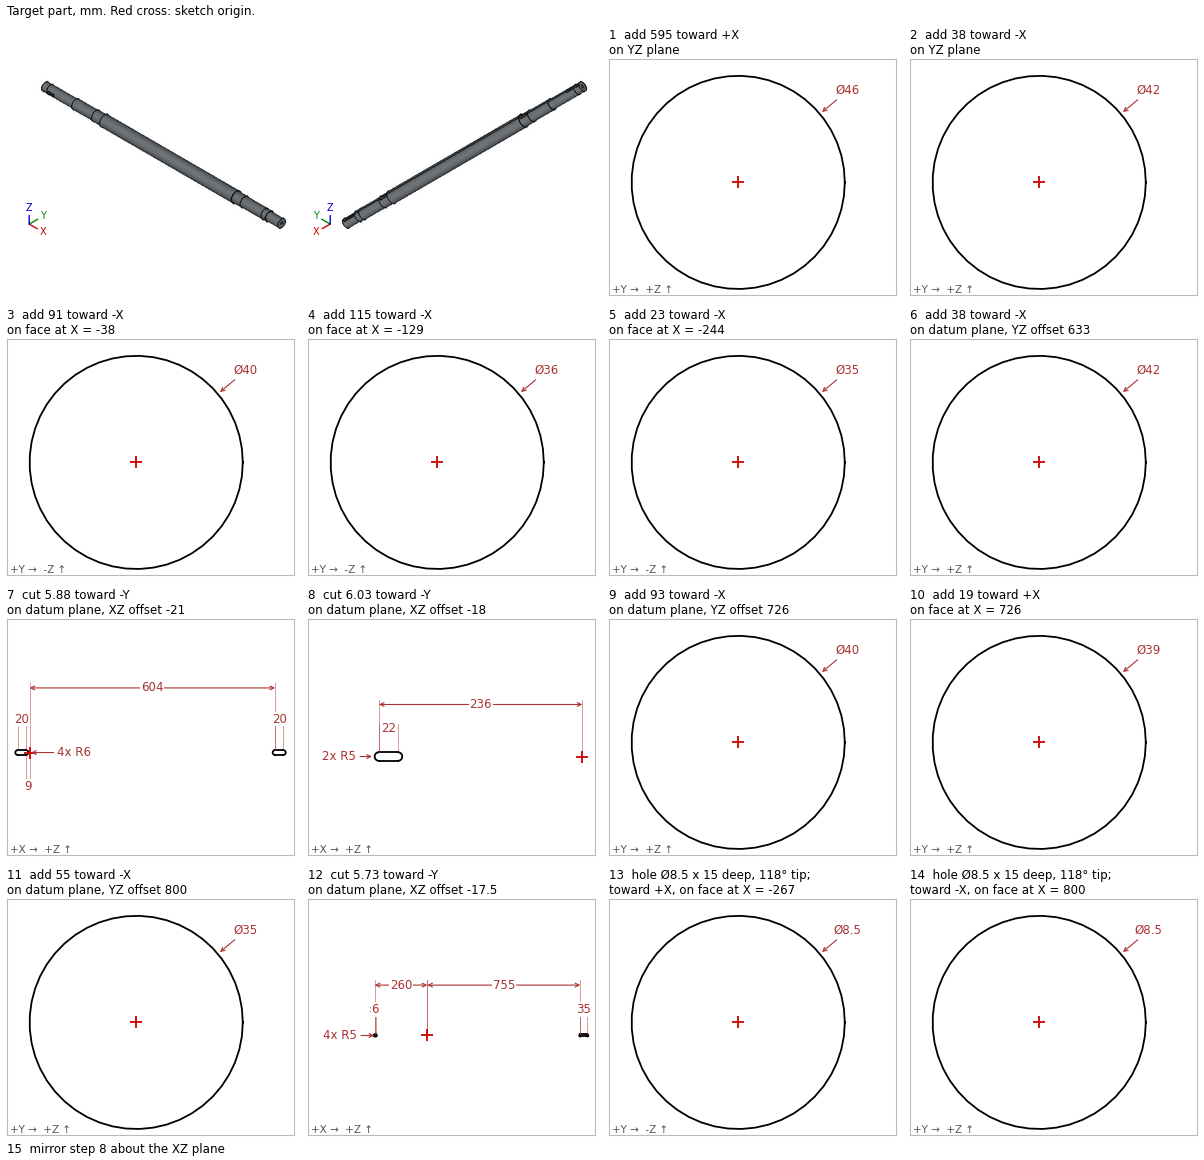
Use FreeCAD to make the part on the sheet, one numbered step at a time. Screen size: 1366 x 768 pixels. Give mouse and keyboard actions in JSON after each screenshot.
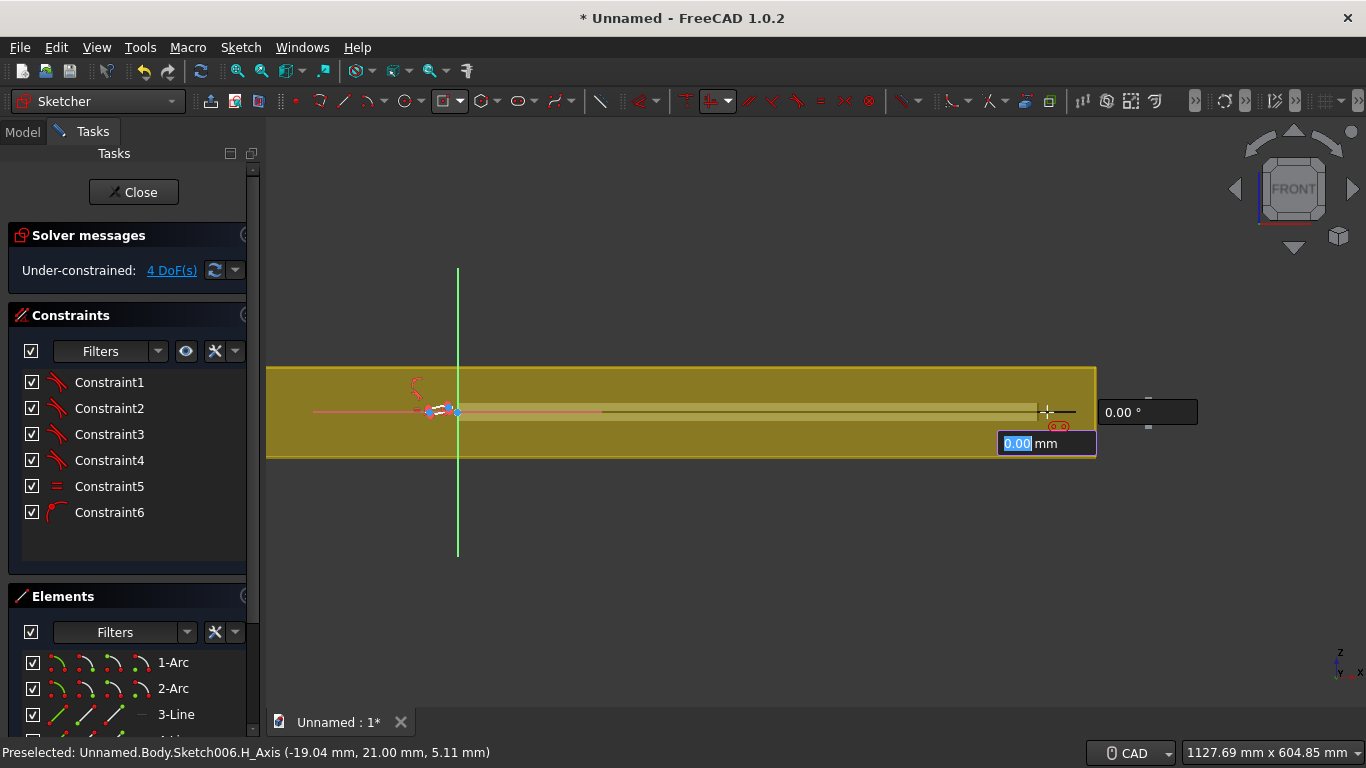
{"action": "left_click", "coordinate": [1066, 403]}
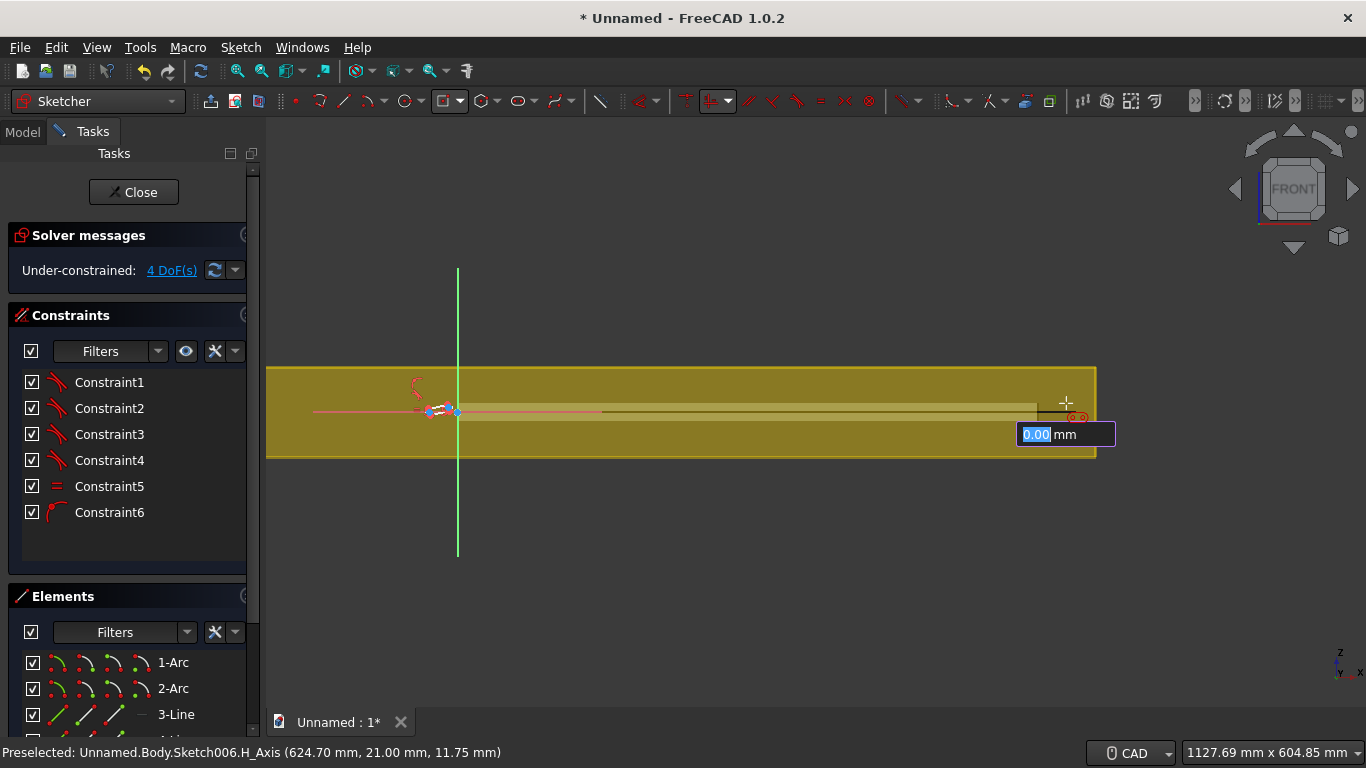
{"action": "scroll", "coordinate": [1057, 418], "scroll_direction": "up", "scroll_amount": 5}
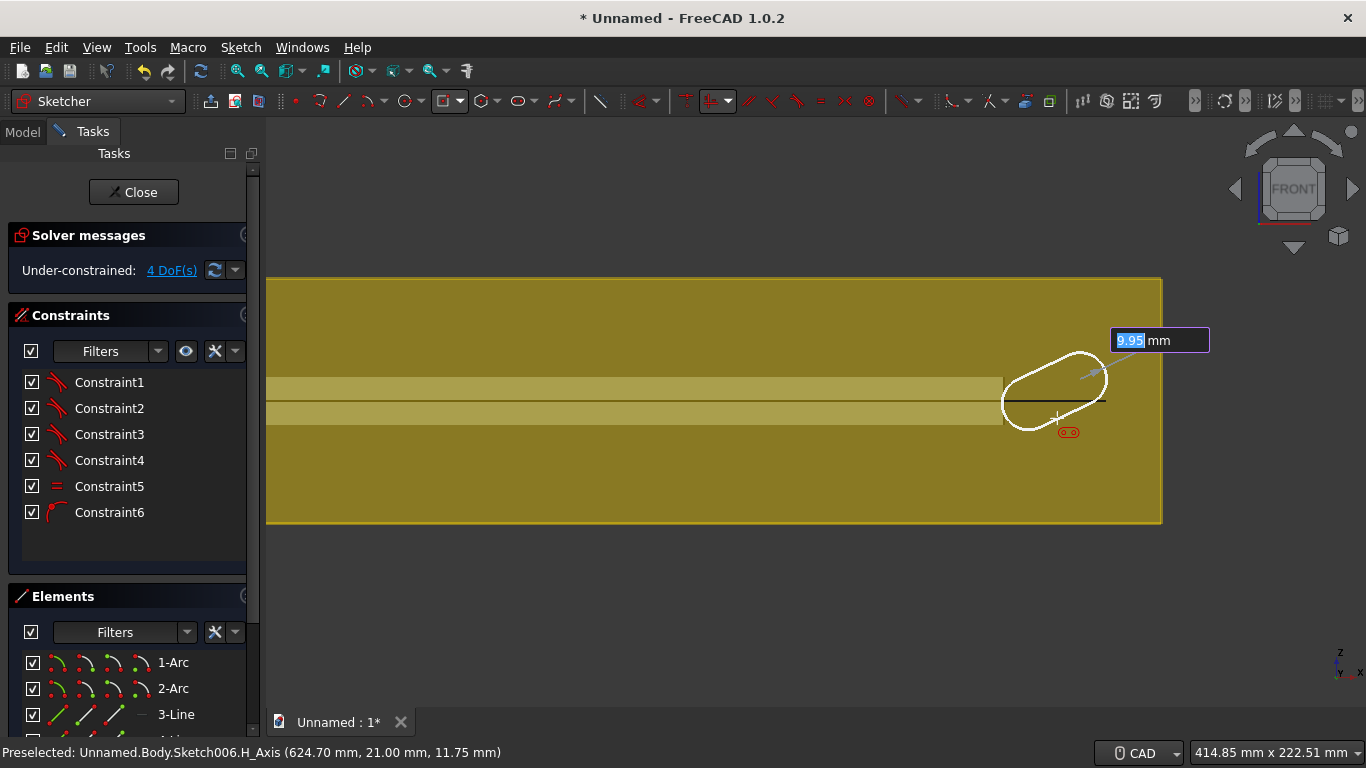
{"action": "left_click", "coordinate": [1055, 417]}
{"action": "key", "text": "Escape"}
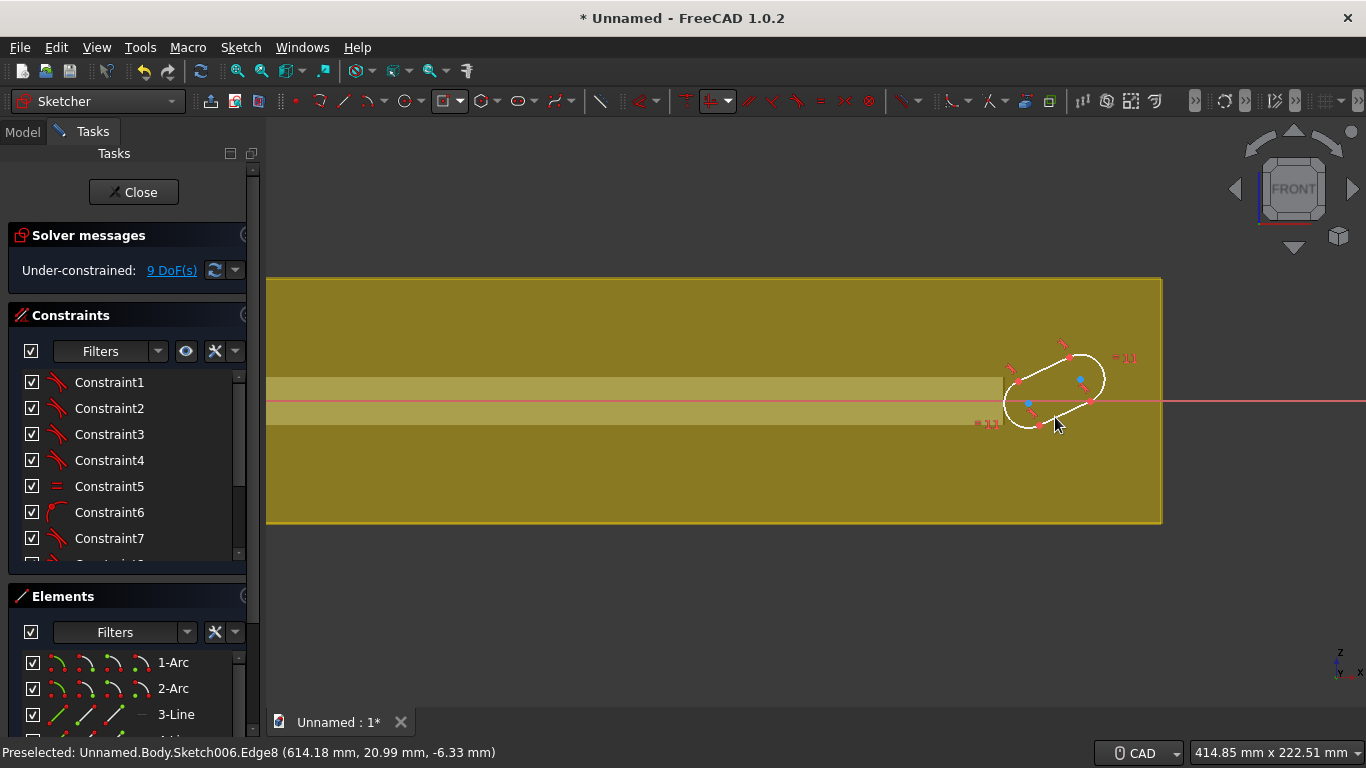
{"action": "scroll", "coordinate": [1057, 418], "scroll_direction": "down", "scroll_amount": 5}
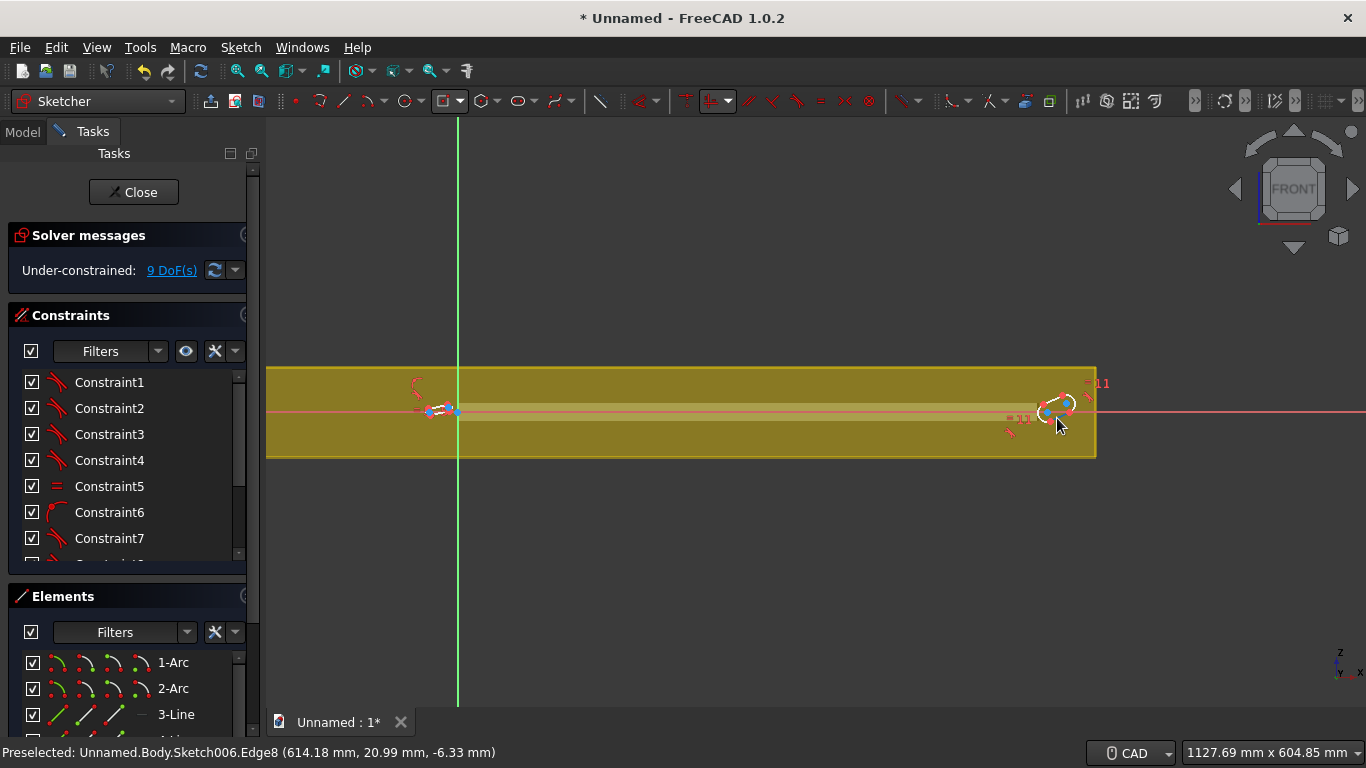
{"action": "scroll", "coordinate": [435, 408], "scroll_direction": "up", "scroll_amount": 6}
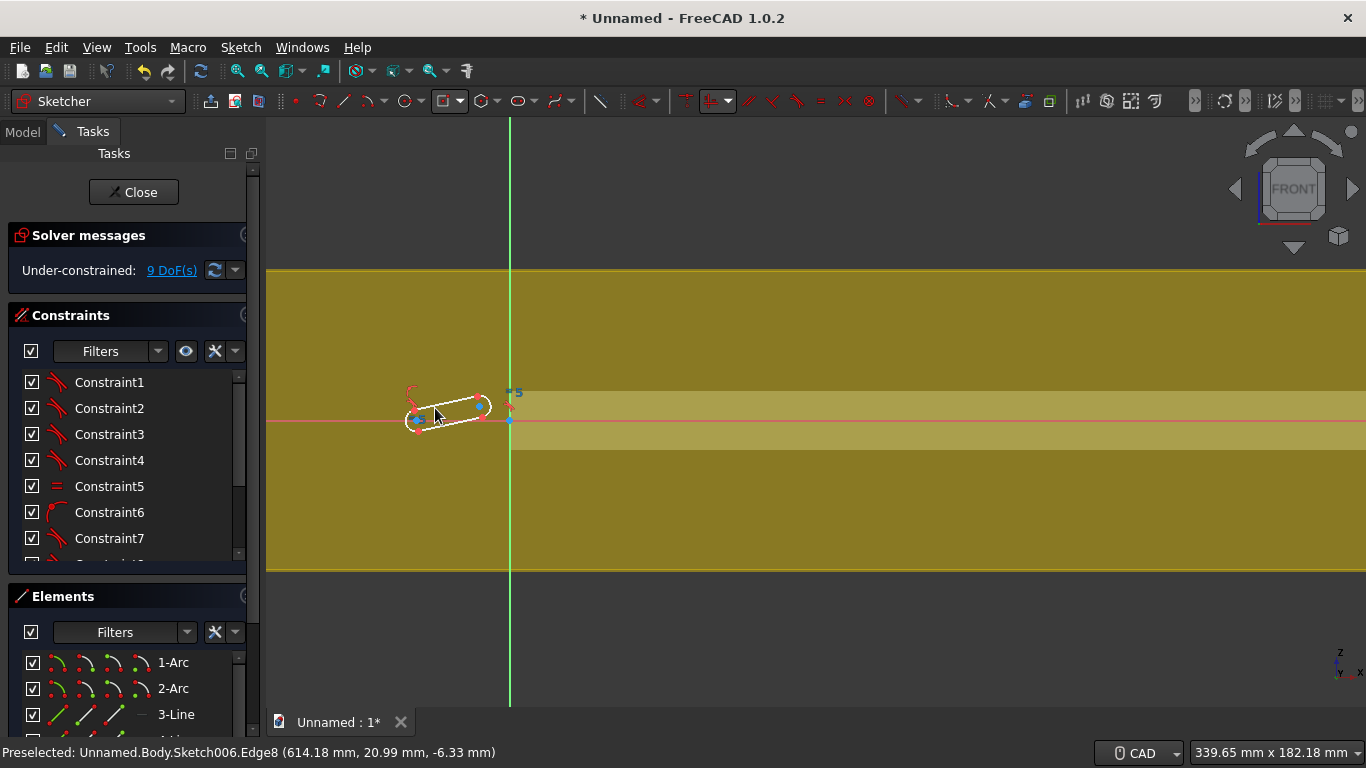
{"action": "left_click", "coordinate": [433, 406]}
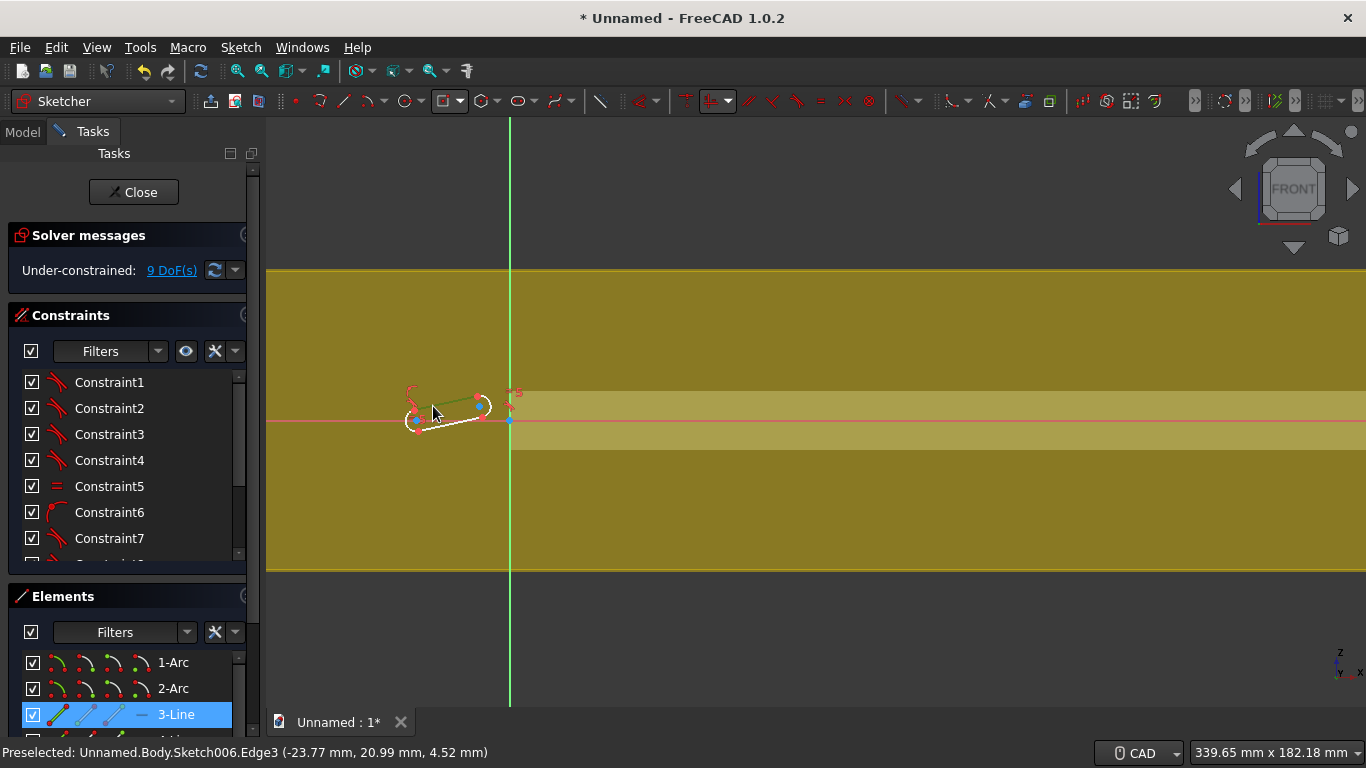
{"action": "key", "text": "h"}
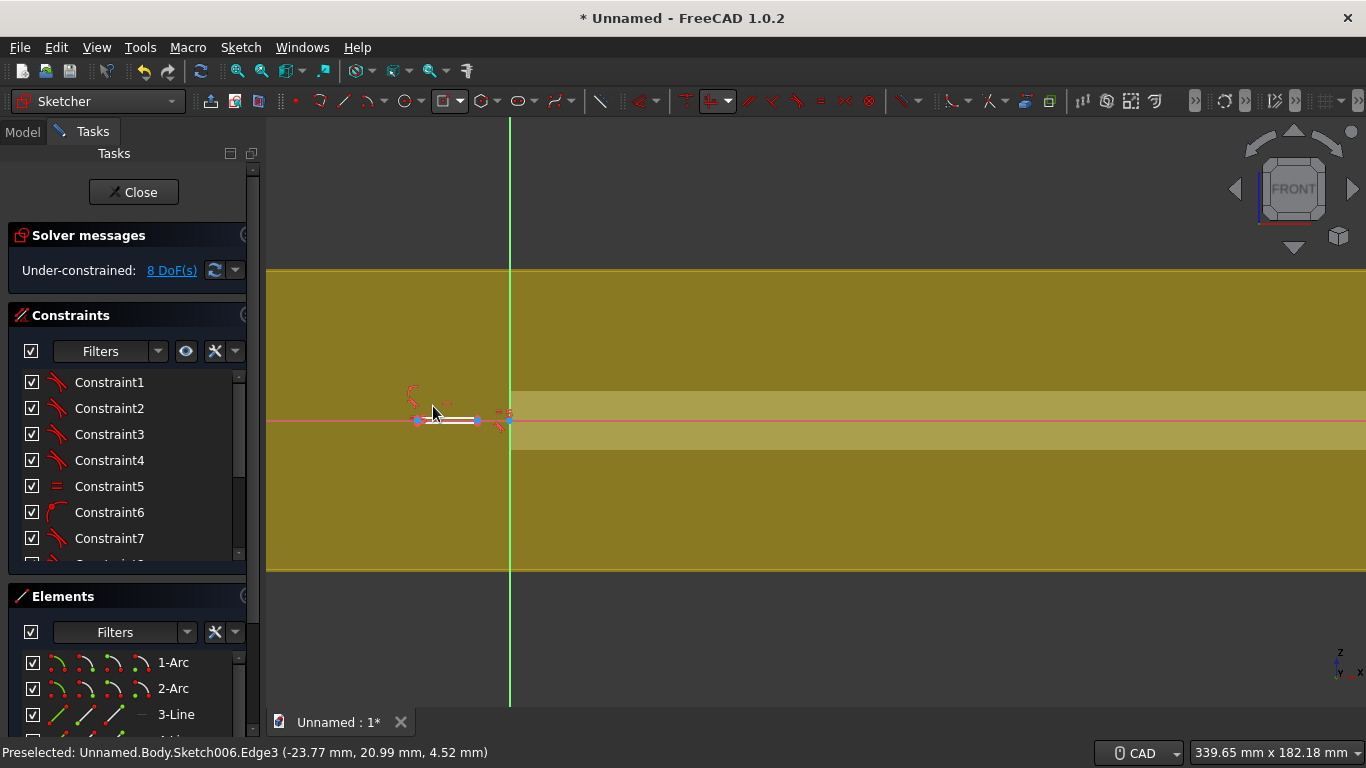
{"action": "scroll", "coordinate": [435, 408], "scroll_direction": "down", "scroll_amount": 6}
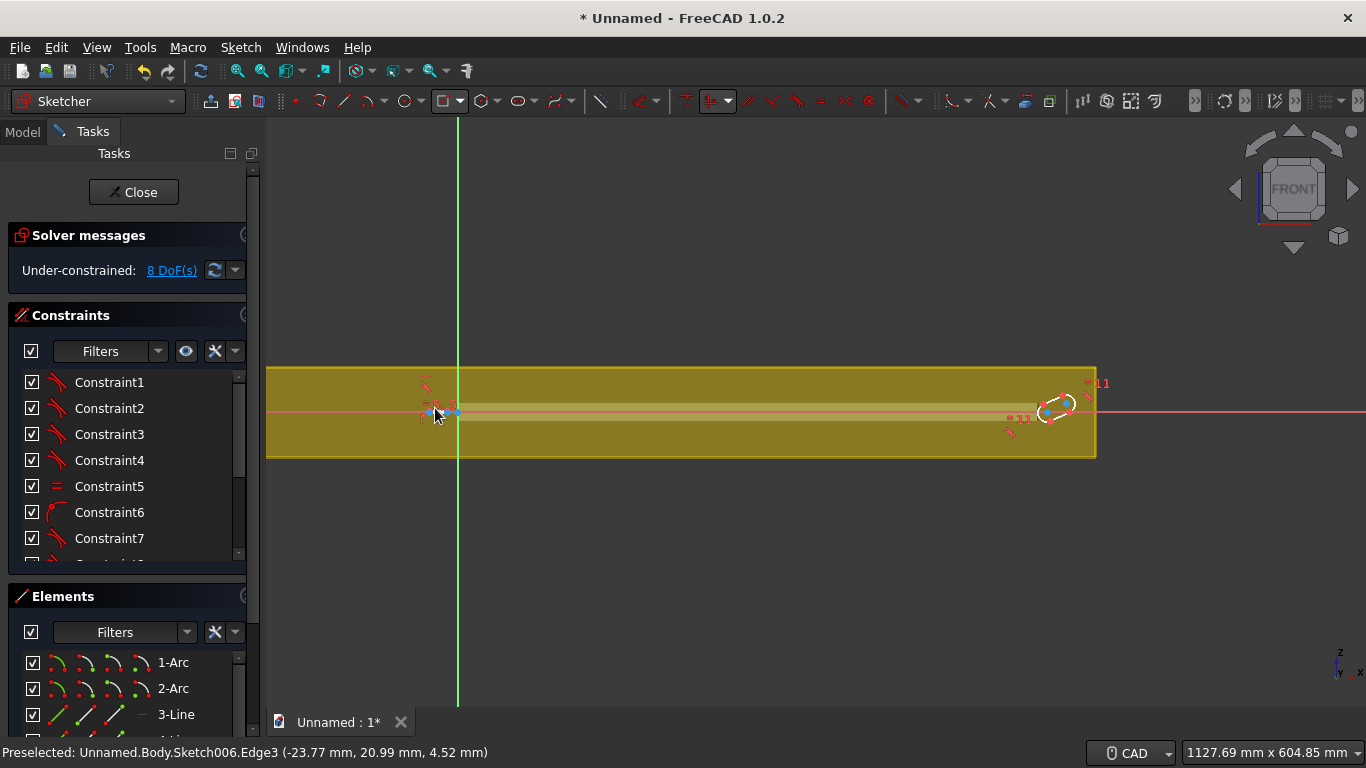
{"action": "scroll", "coordinate": [1049, 402], "scroll_direction": "up", "scroll_amount": 4}